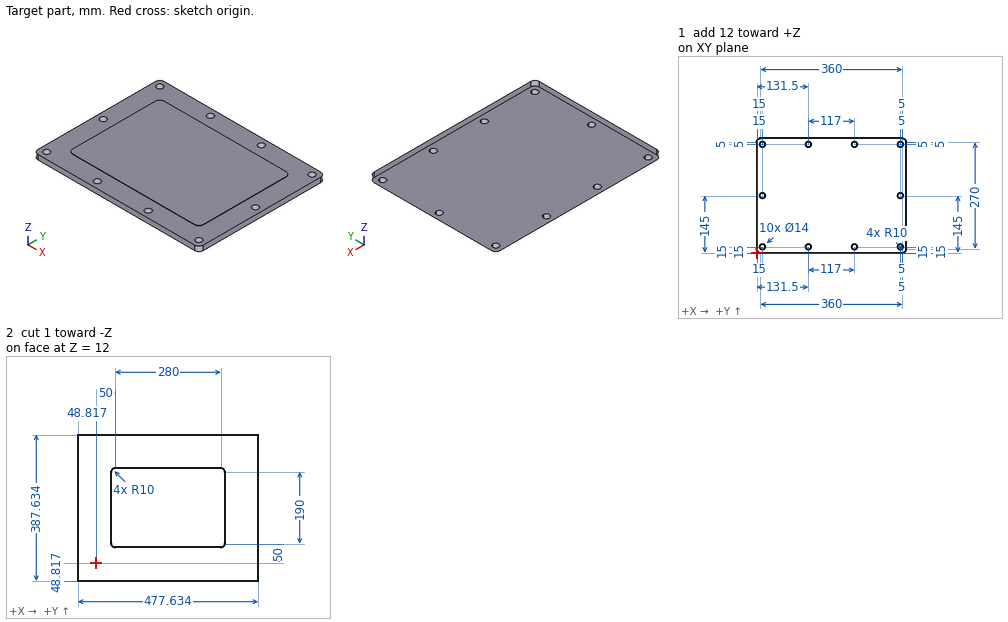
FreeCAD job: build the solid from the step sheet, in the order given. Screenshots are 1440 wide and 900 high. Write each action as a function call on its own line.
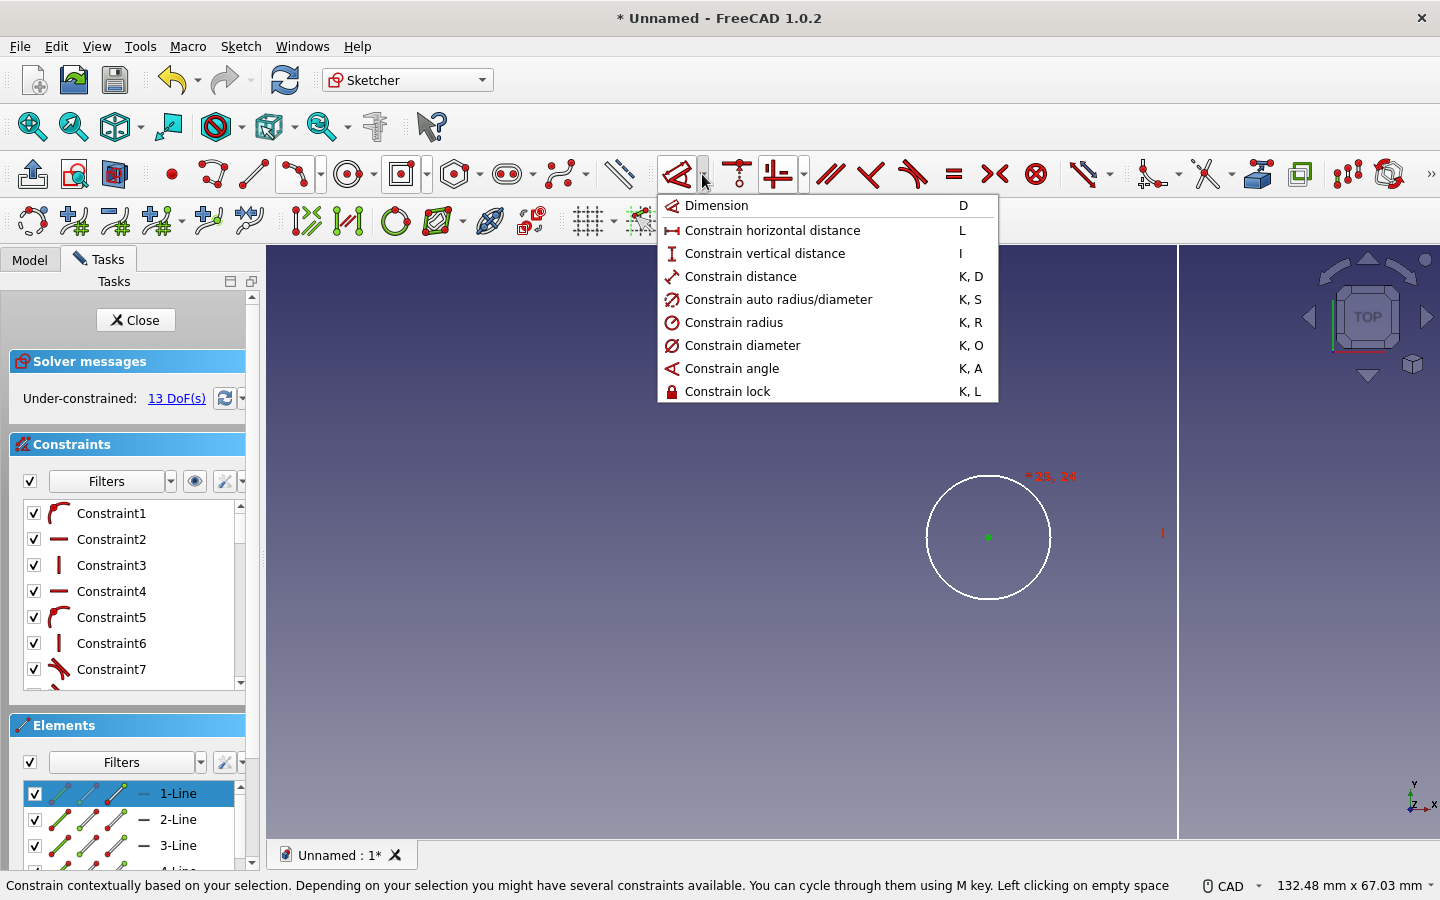
click(828, 230)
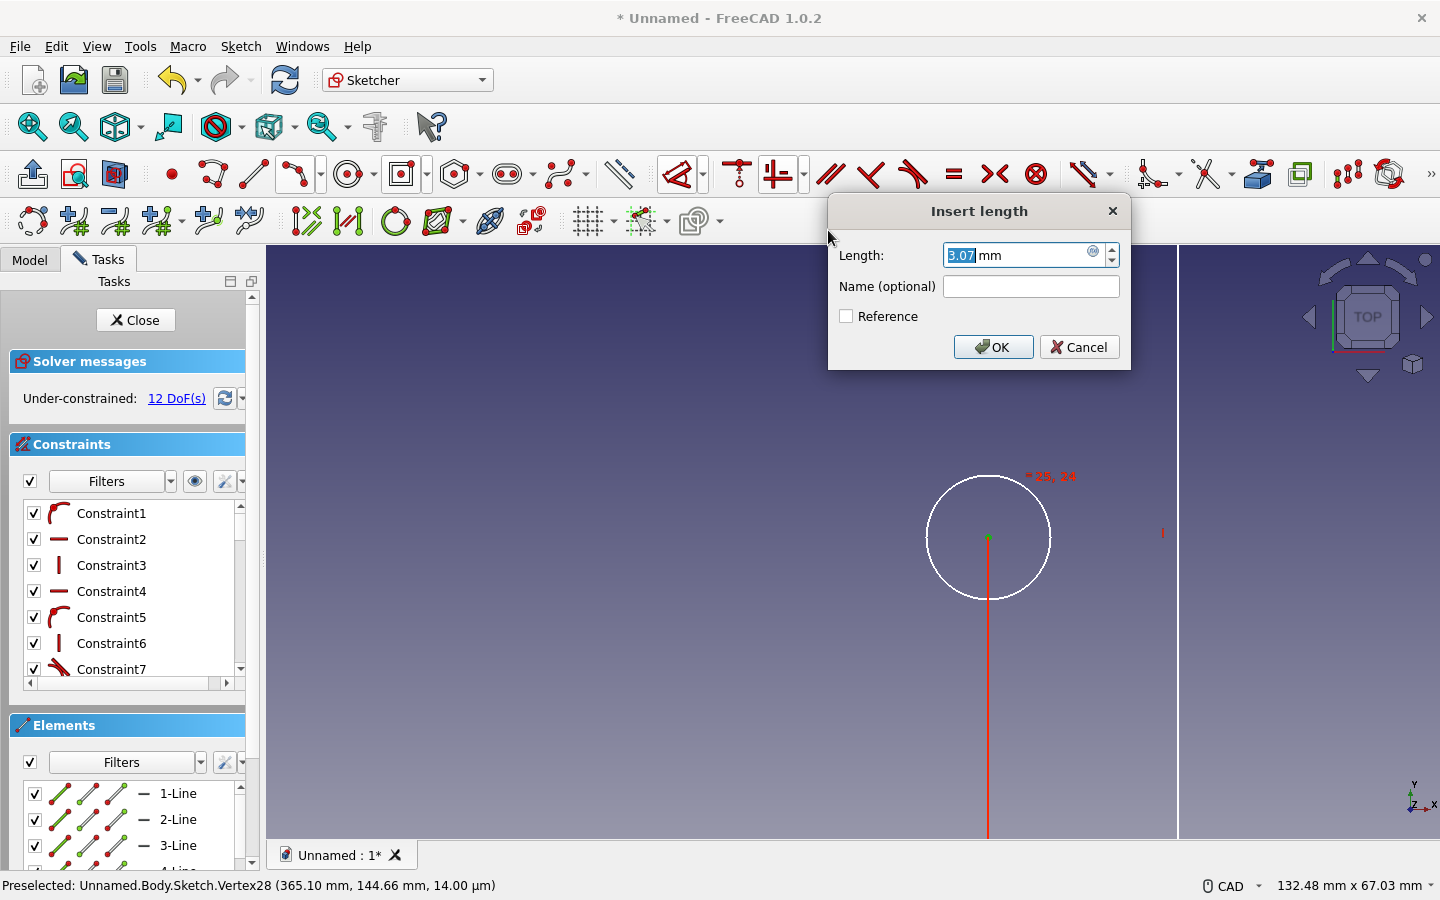
text(5)
key(Return)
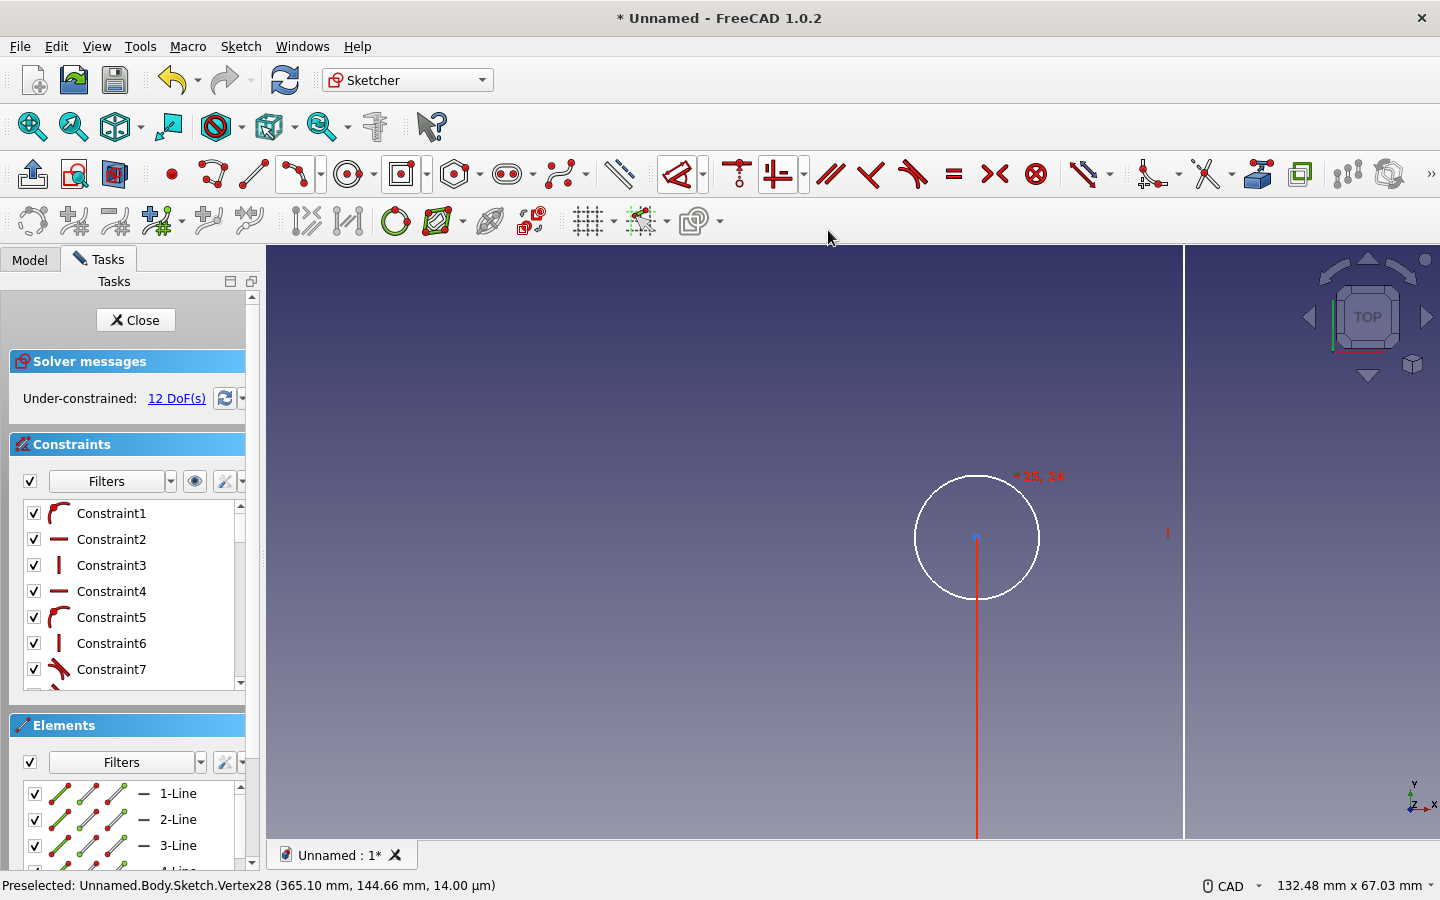
scroll(995, 543, down, 10)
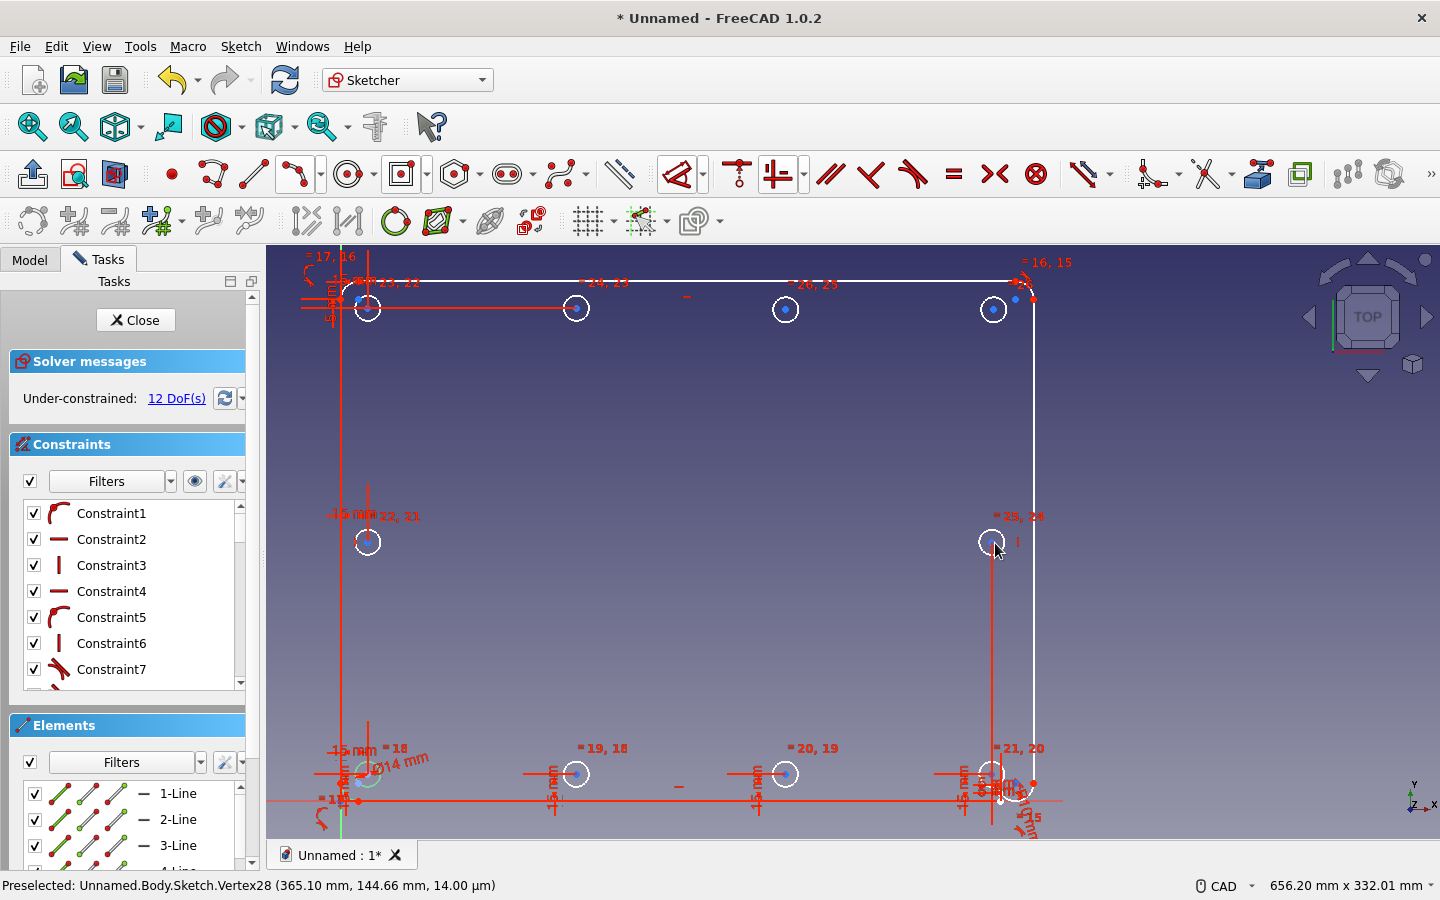
scroll(1021, 380, up, 10)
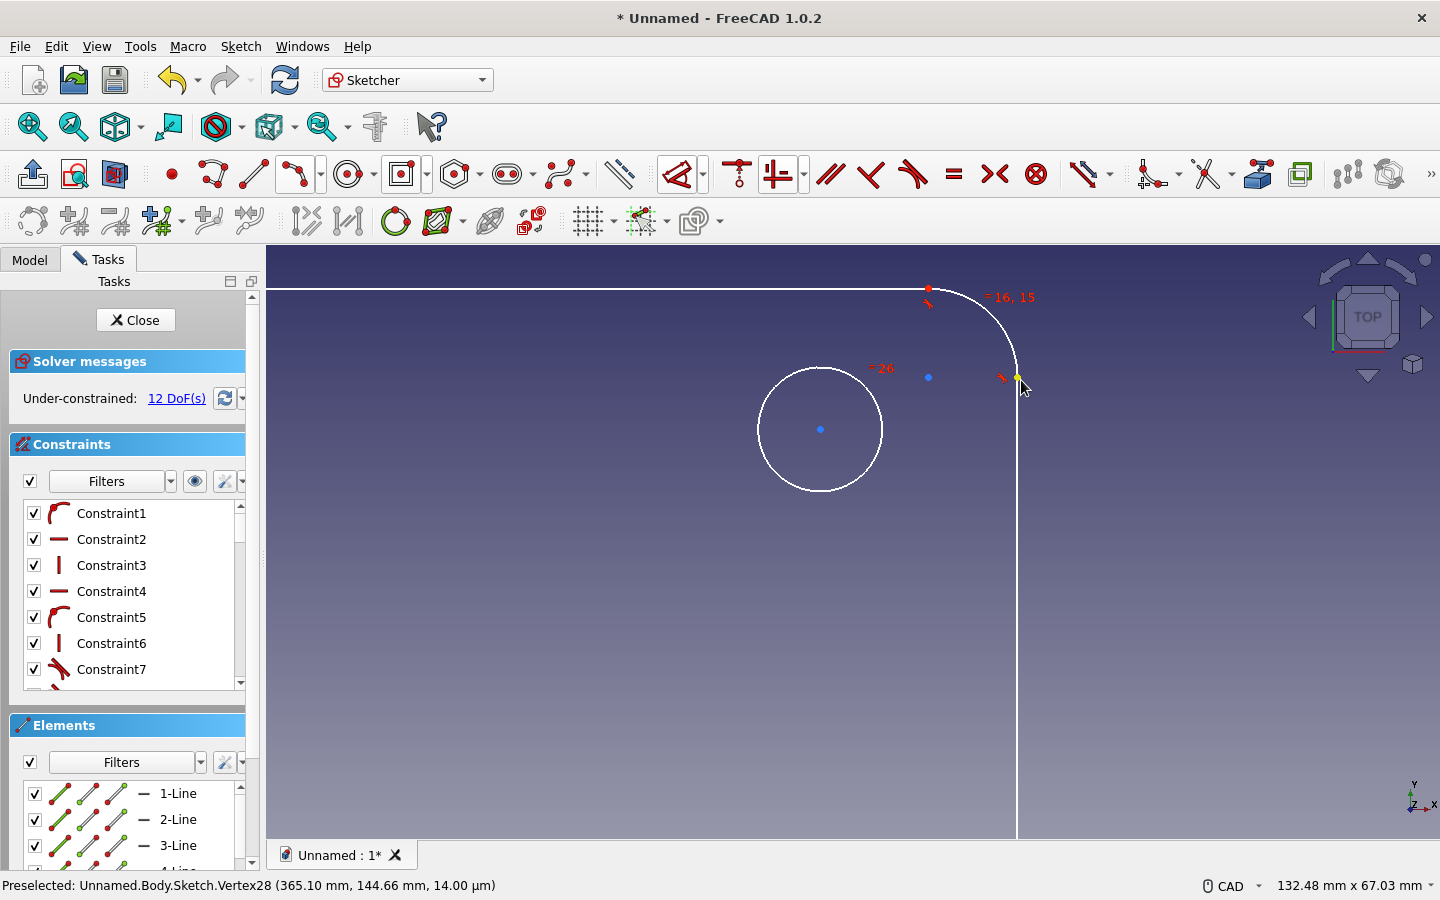
click(1017, 377)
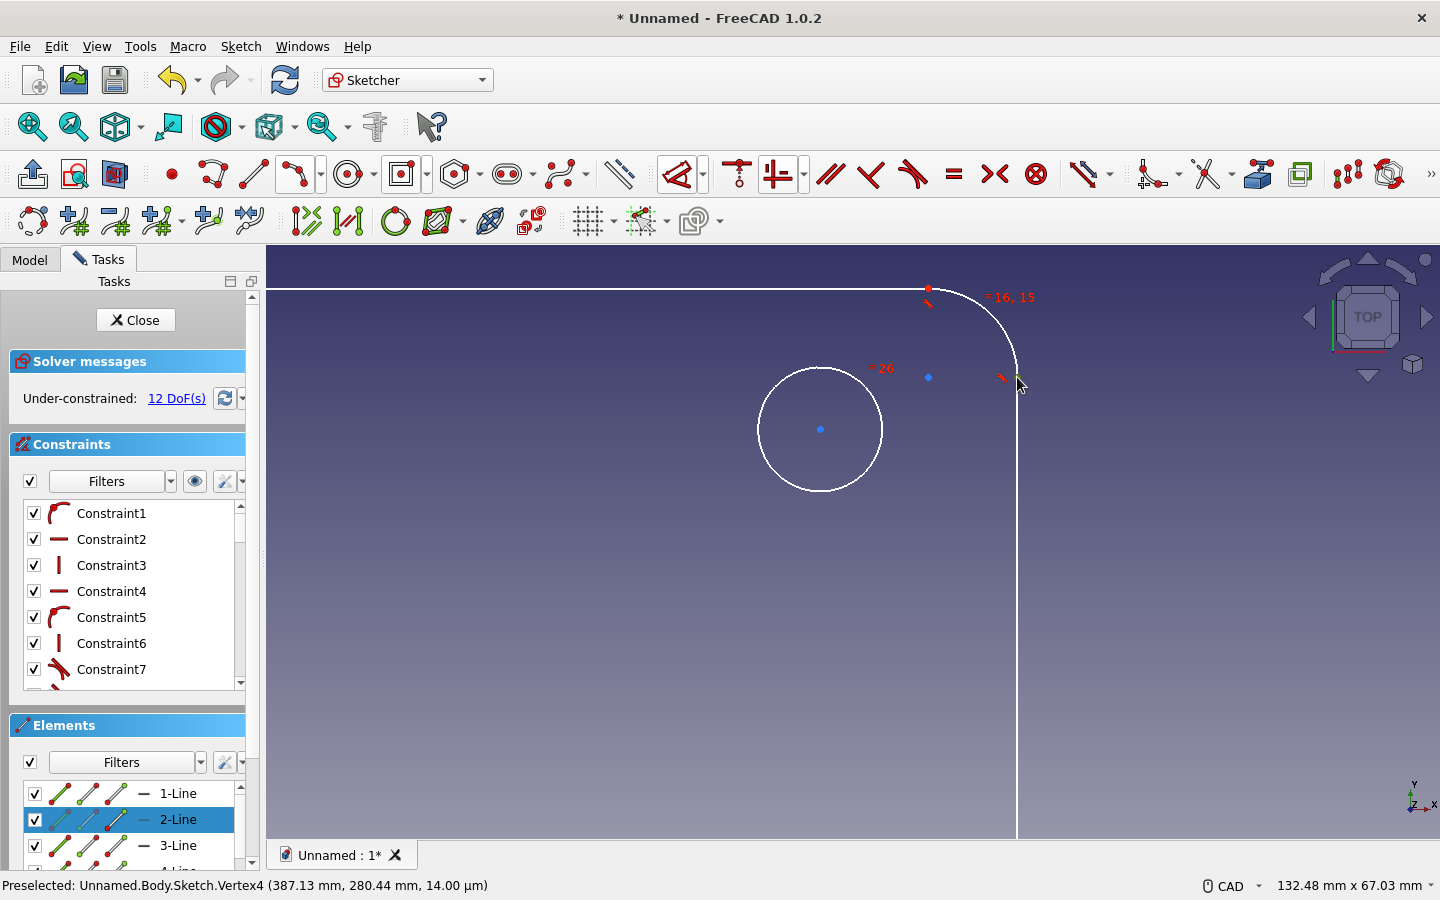
scroll(1021, 380, down, 10)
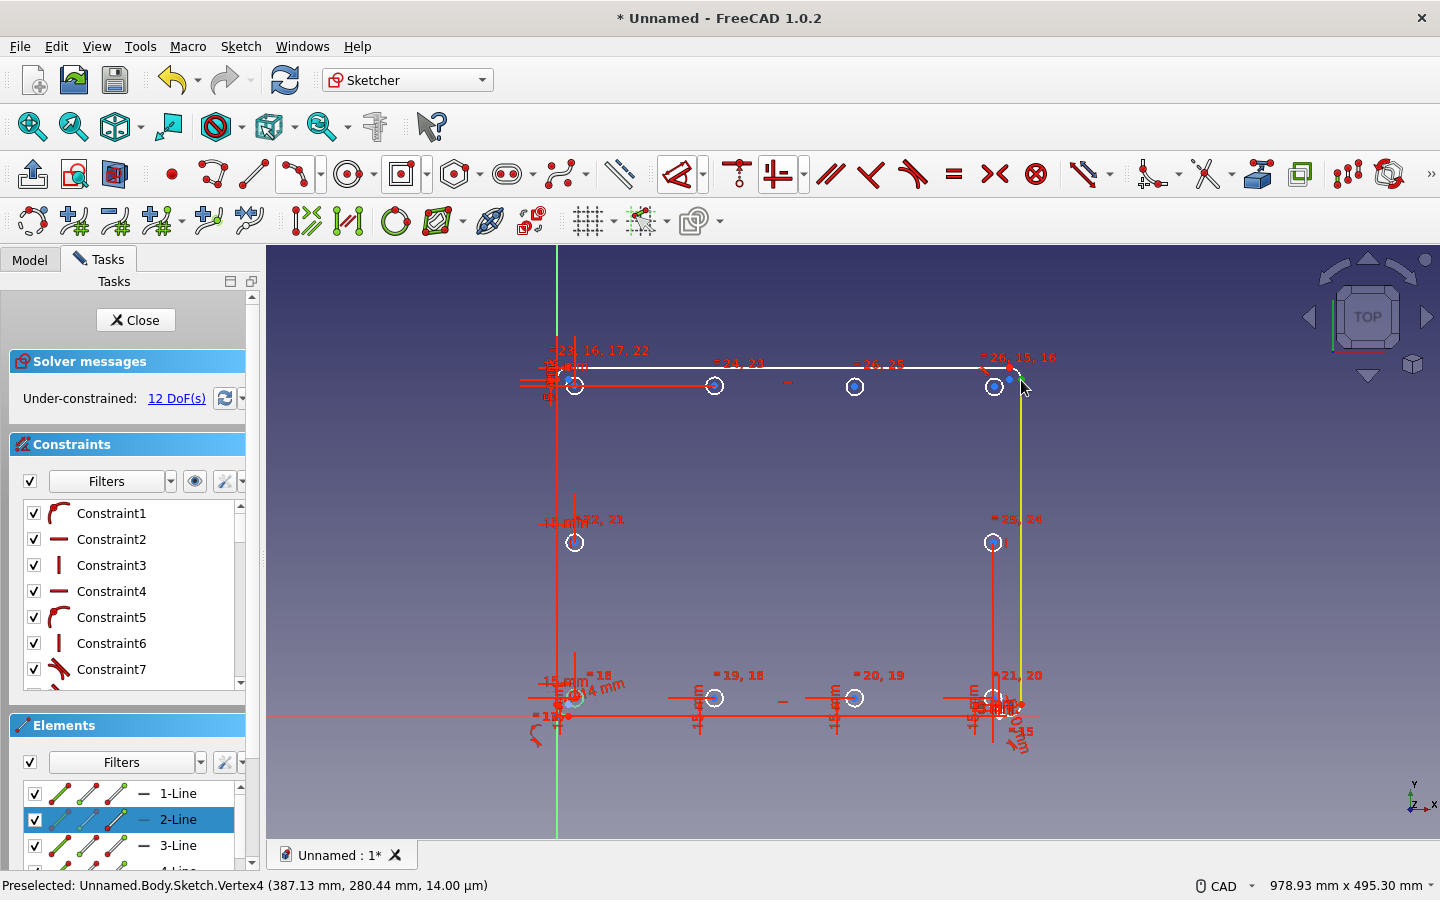
scroll(855, 387, up, 10)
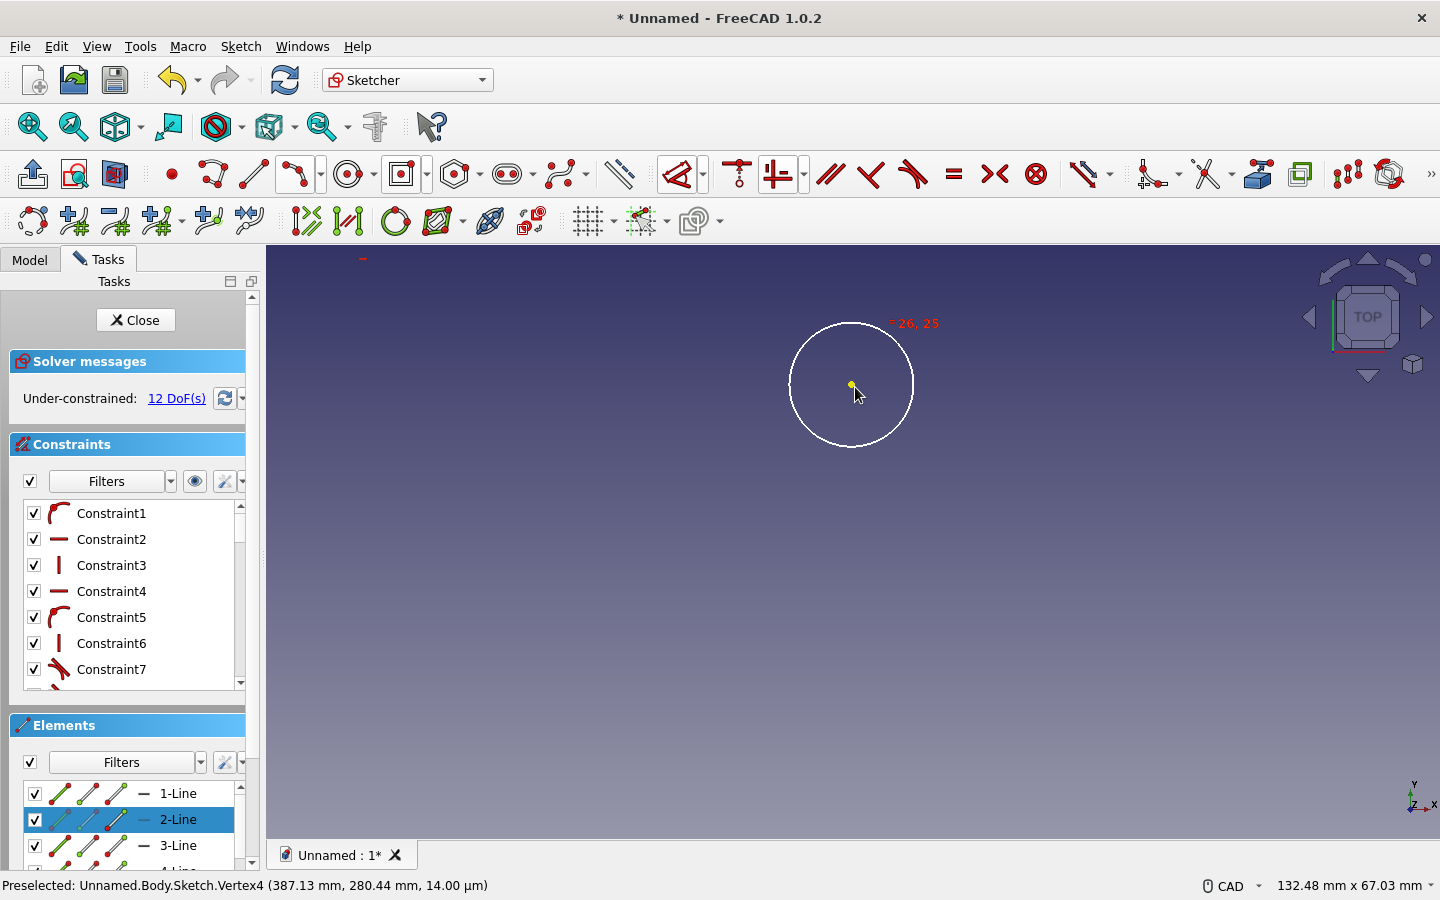
click(851, 385)